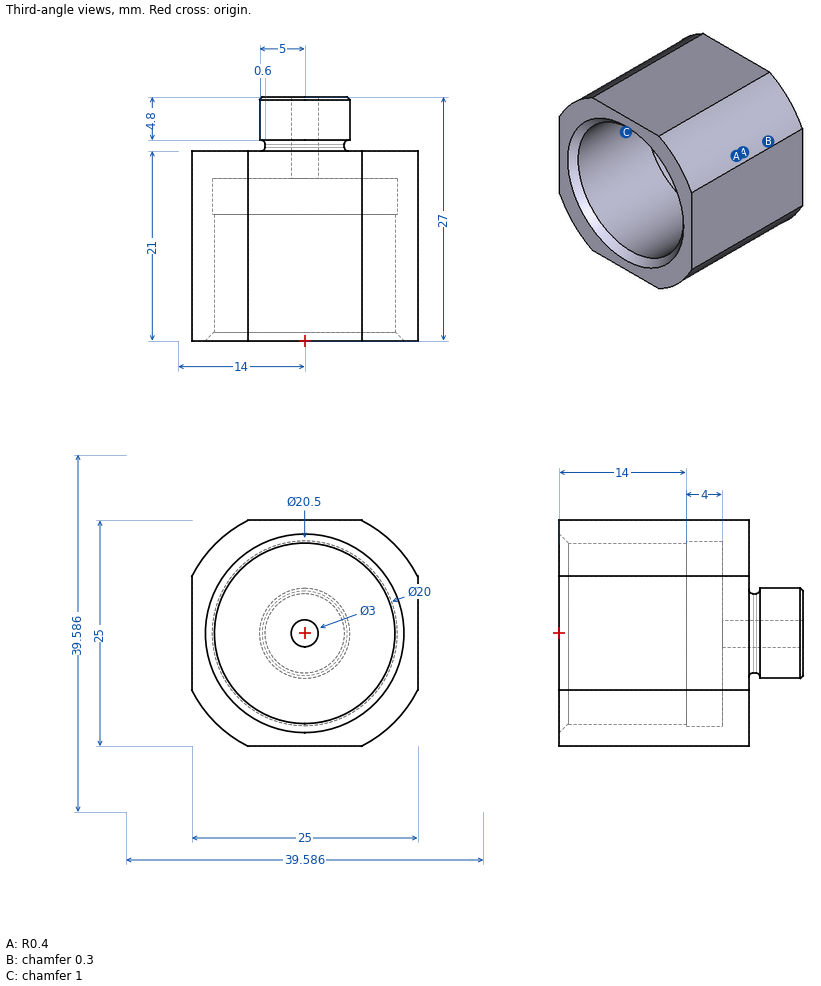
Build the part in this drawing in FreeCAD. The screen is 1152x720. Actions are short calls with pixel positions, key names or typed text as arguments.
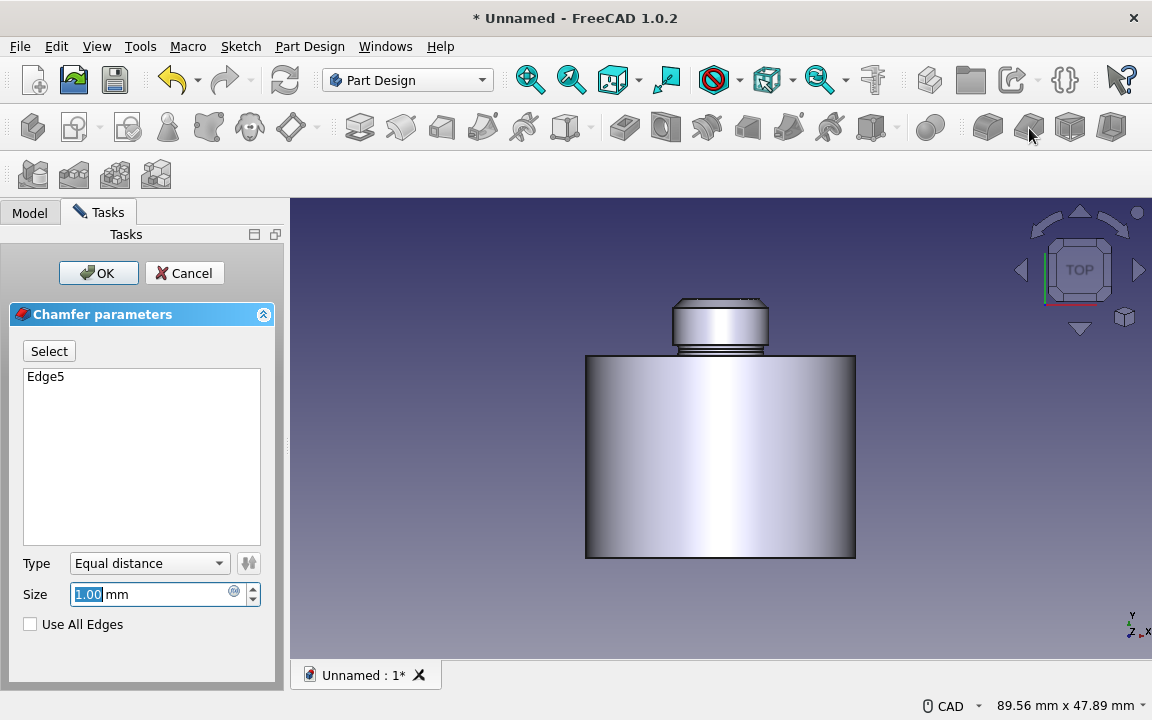
text(0.3)
key(Tab)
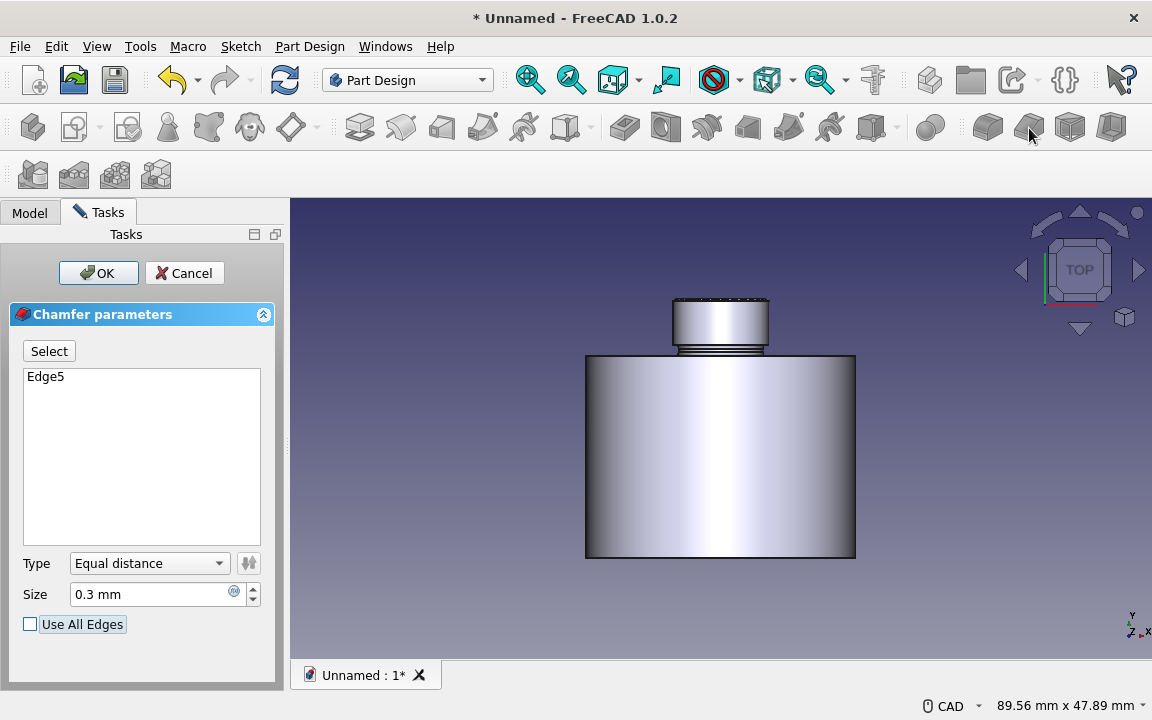
click(99, 273)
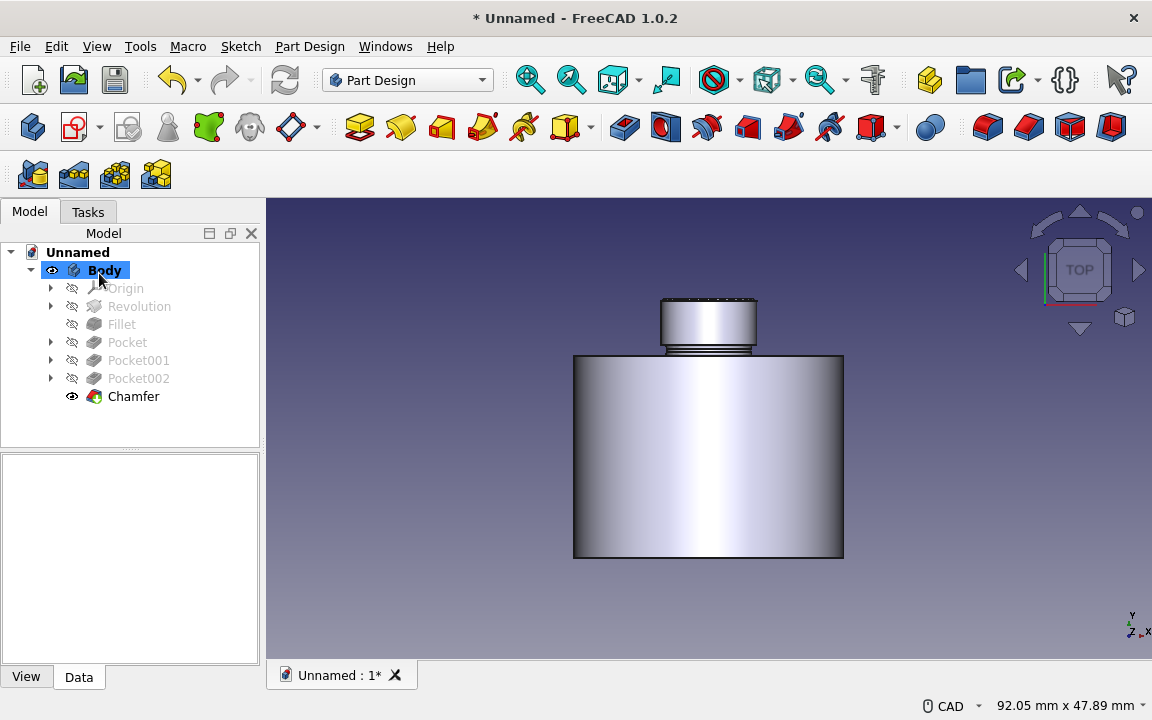
key(0)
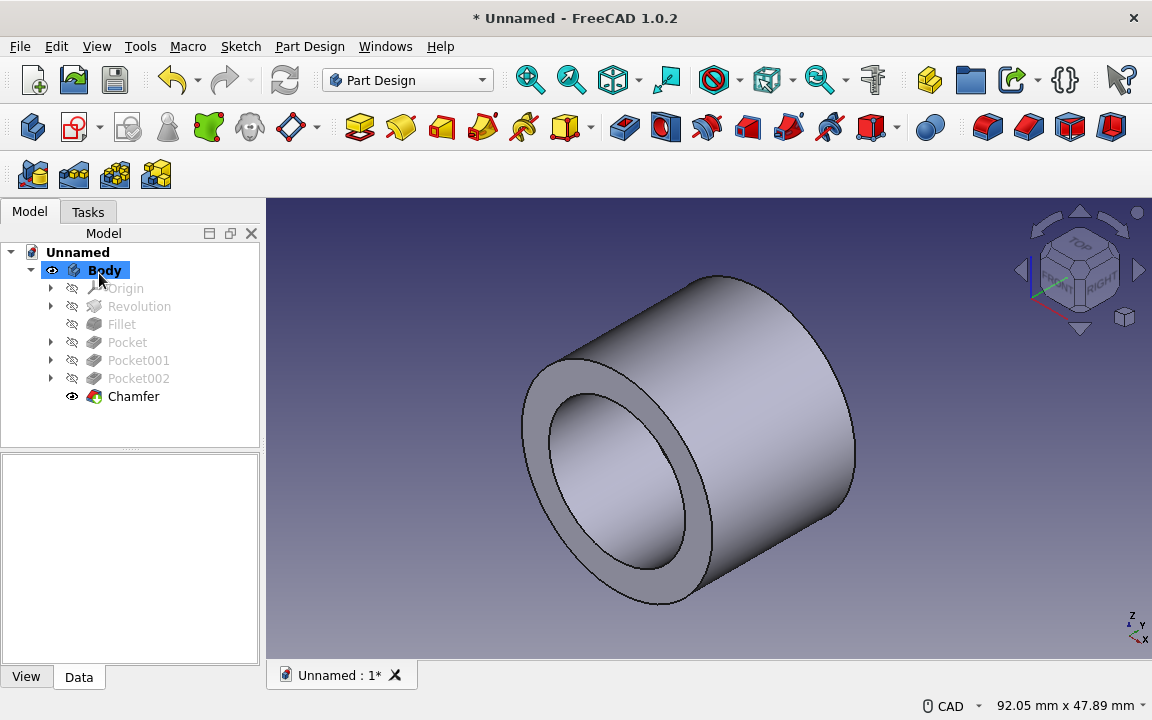
click(549, 441)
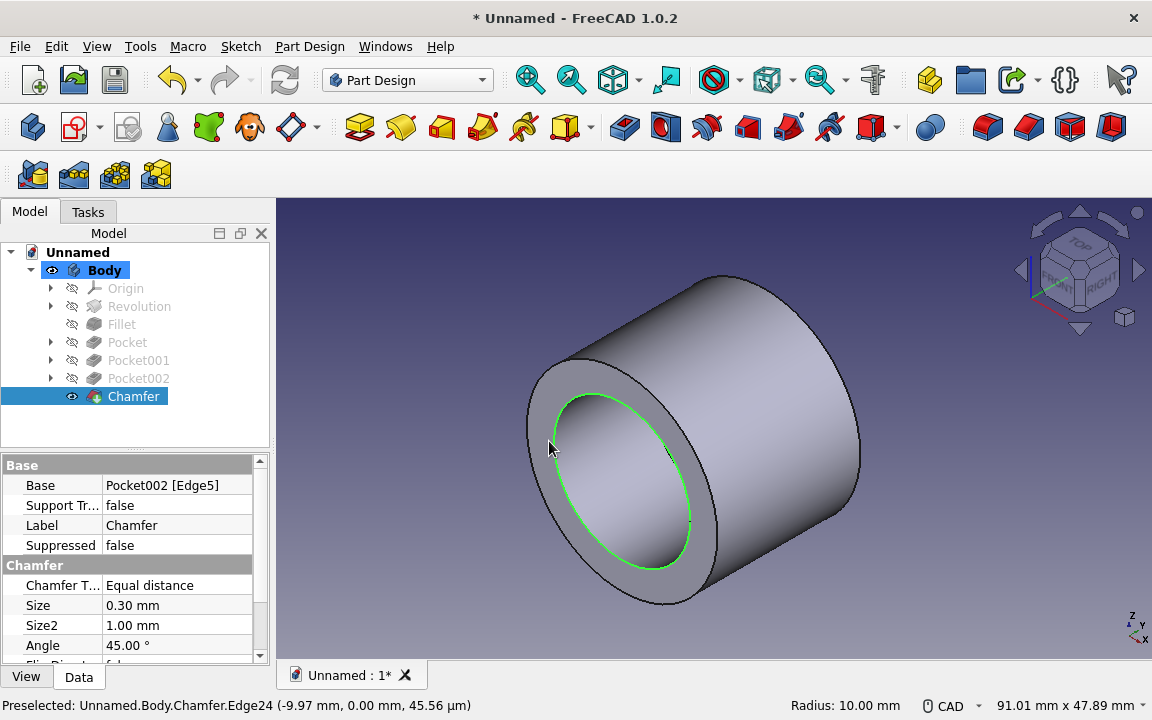
click(1029, 128)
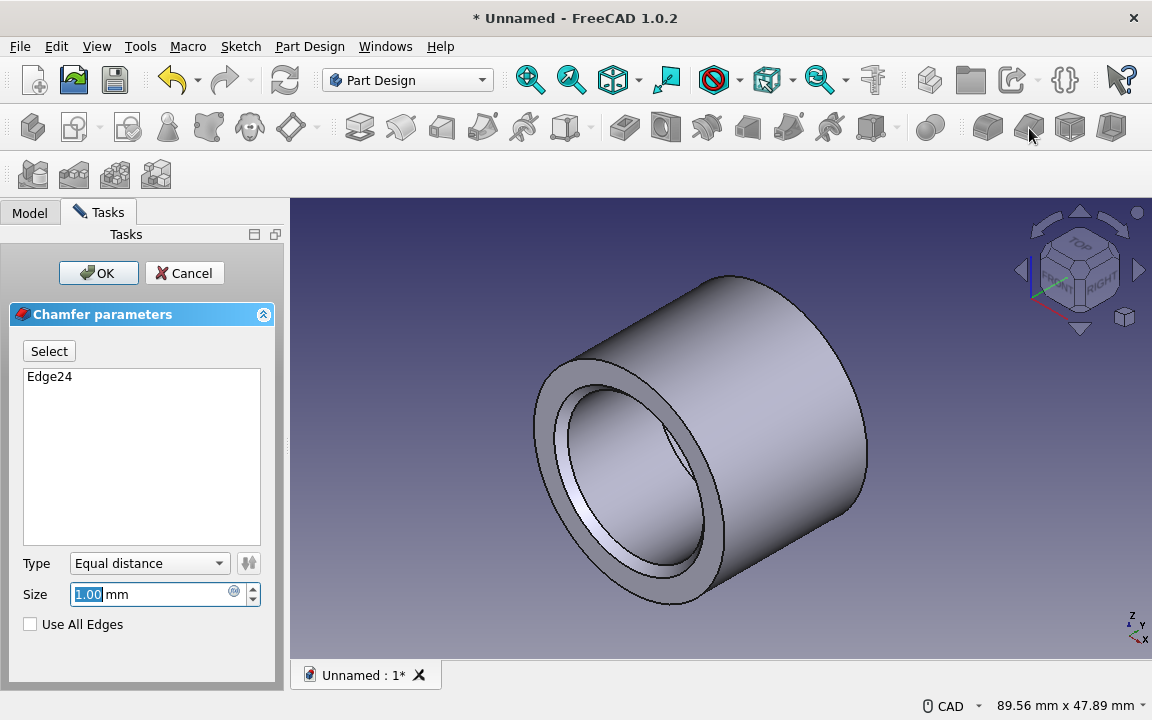
text(1)
key(Tab)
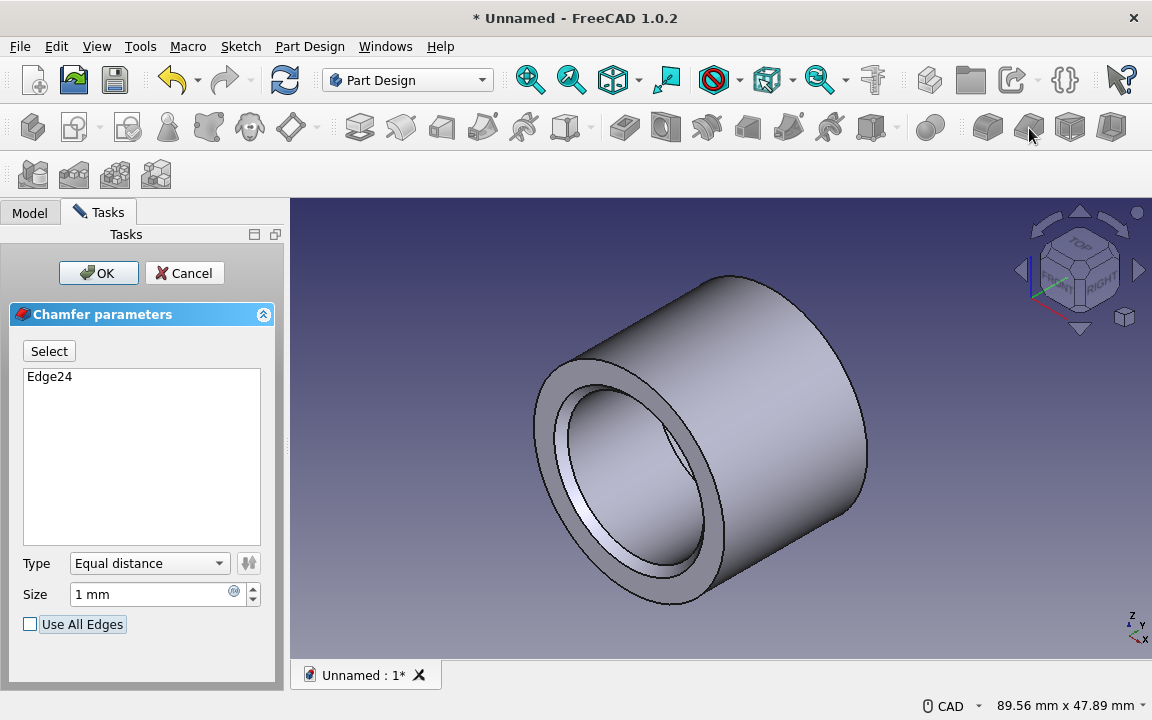
click(99, 273)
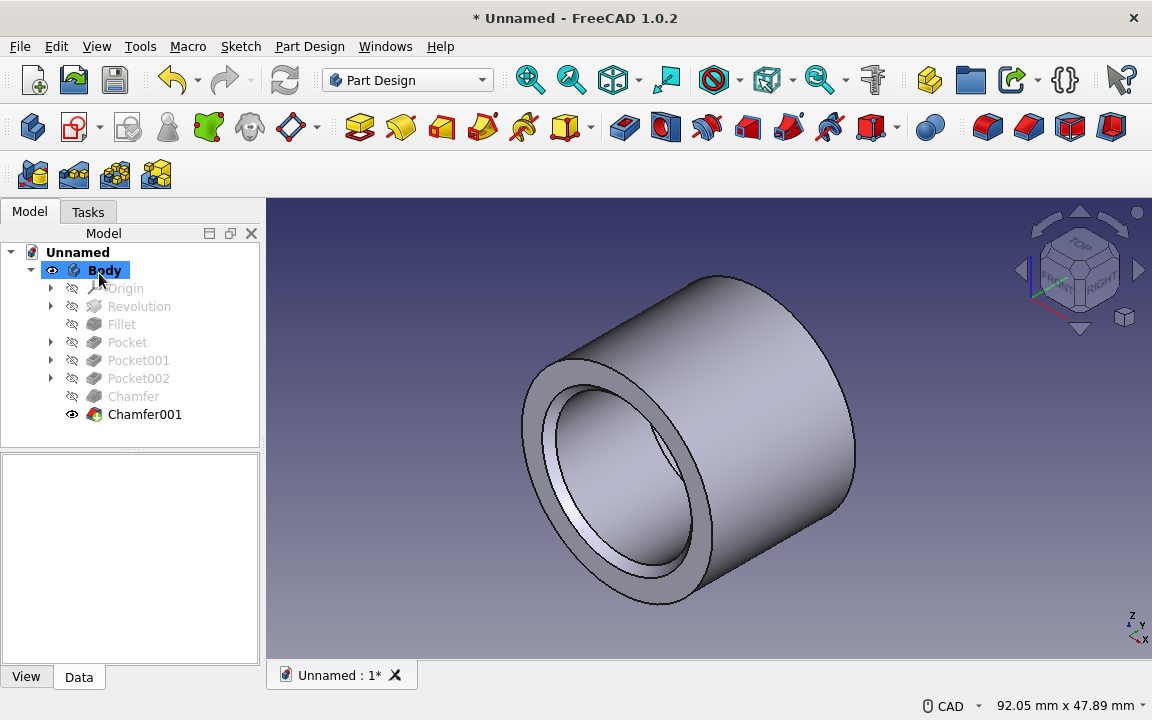
key(4)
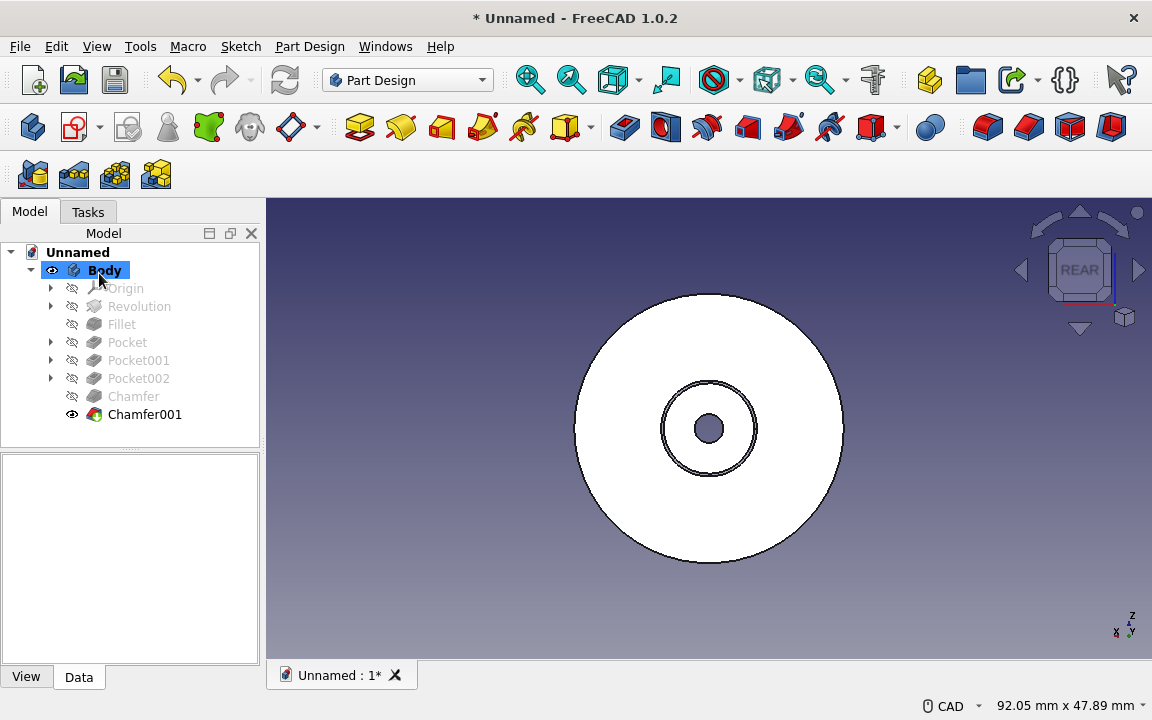
click(632, 389)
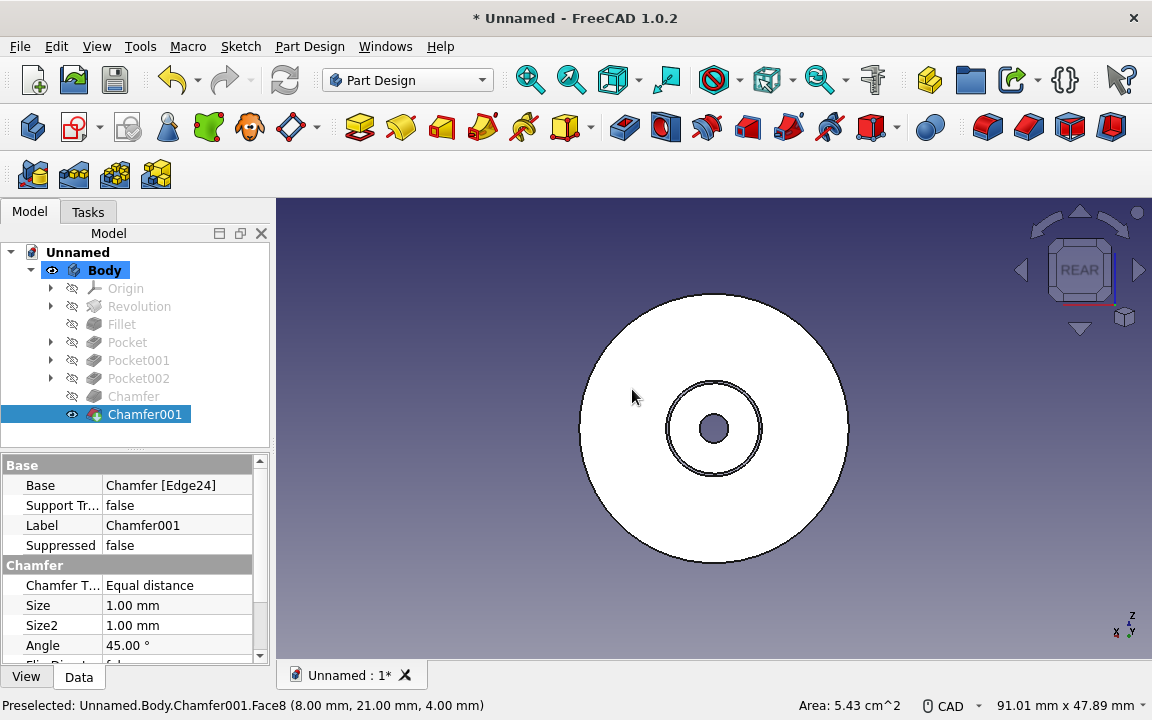
click(74, 128)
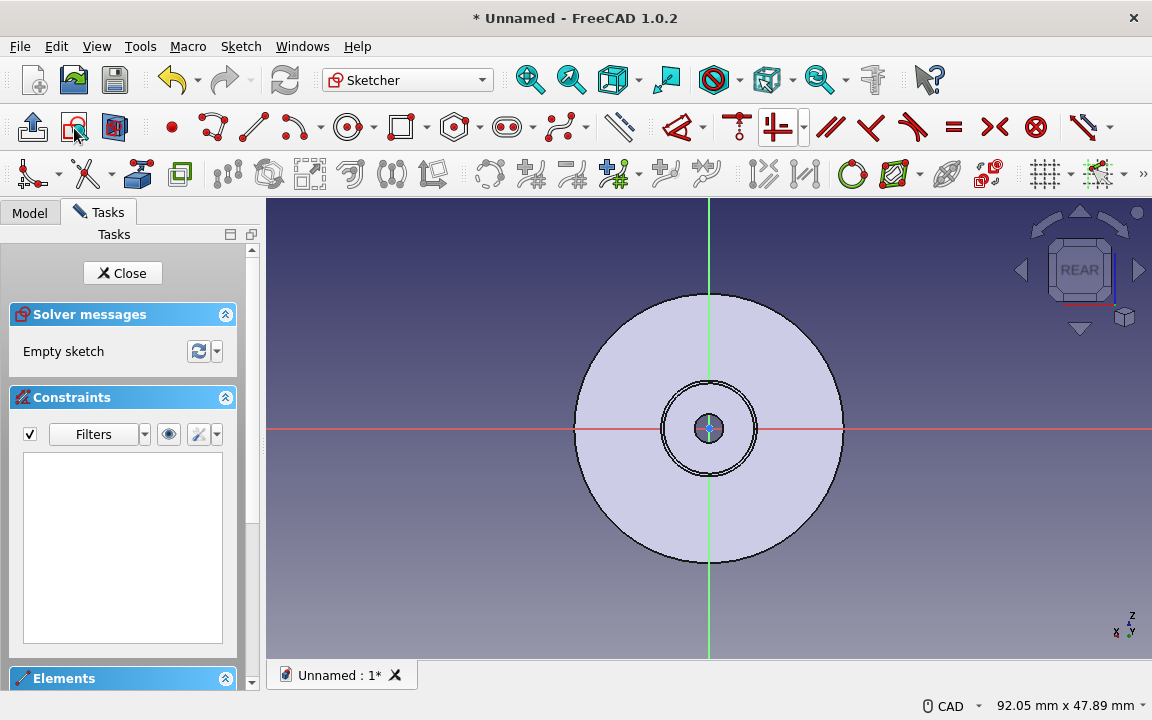
click(115, 128)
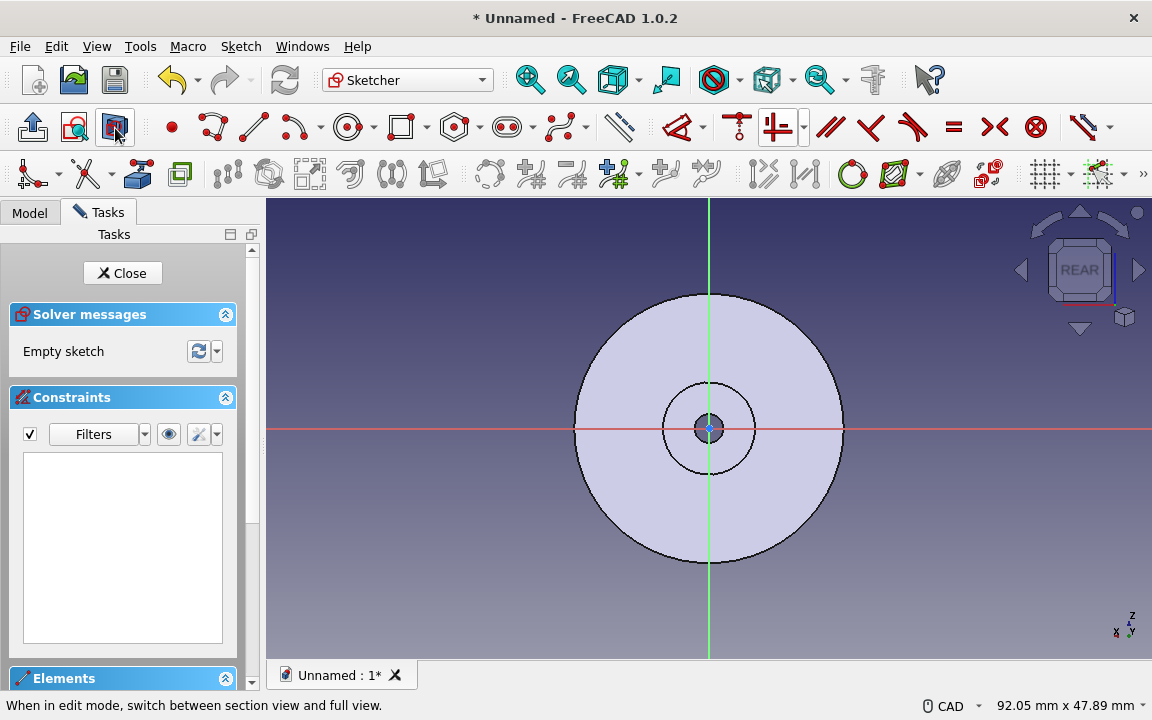
scroll(331, 429, down, 1)